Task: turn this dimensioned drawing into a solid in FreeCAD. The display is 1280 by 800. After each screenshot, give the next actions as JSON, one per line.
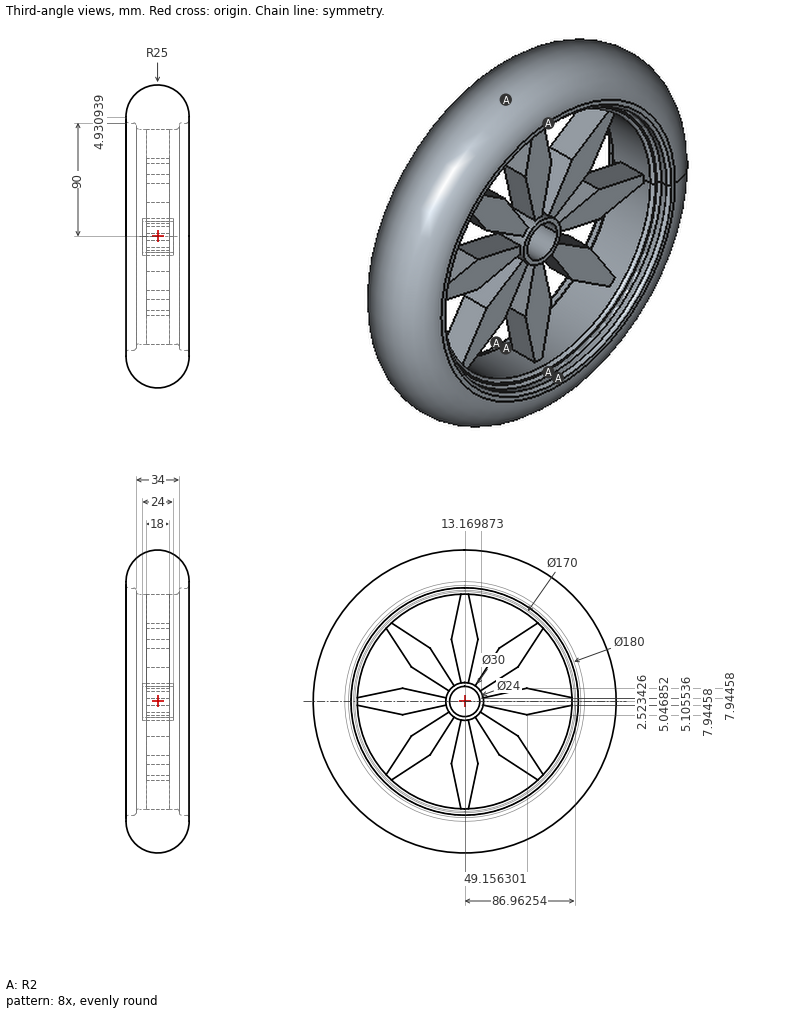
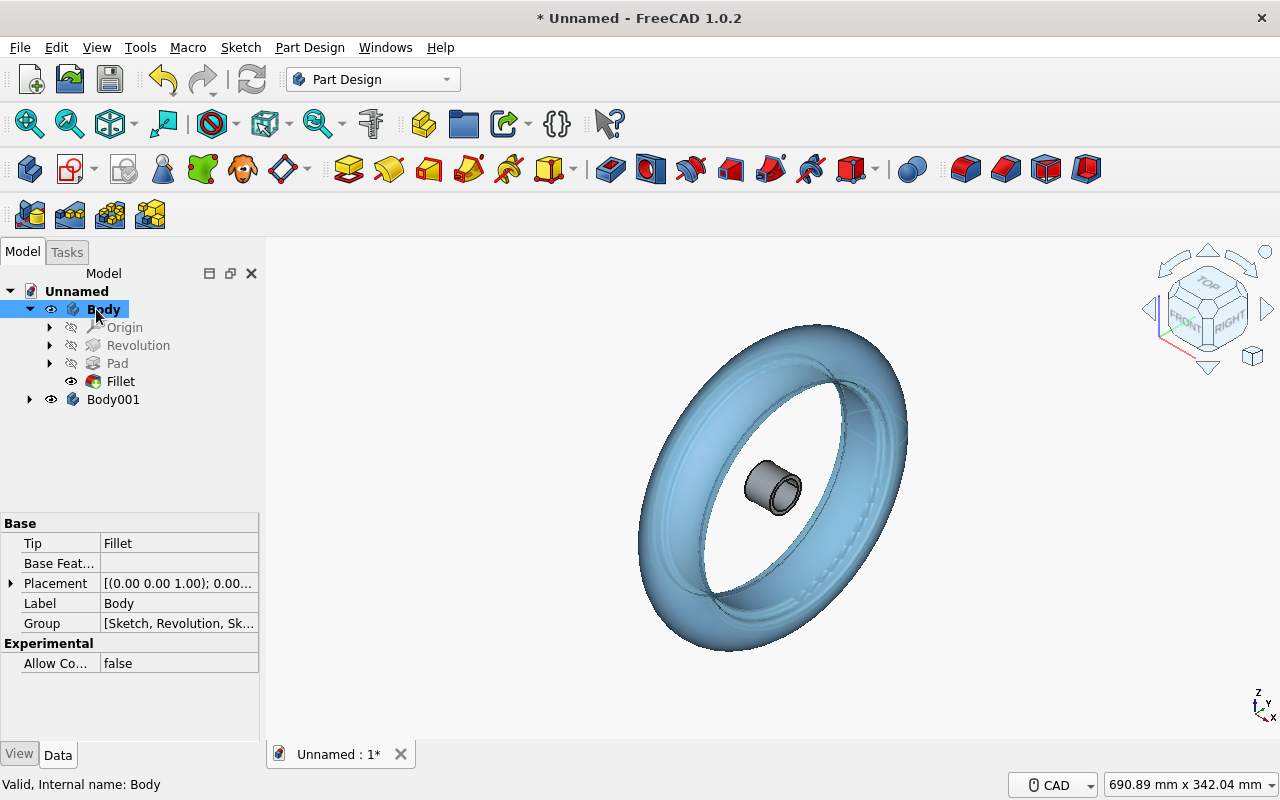
{"action": "left_click", "coordinate": [146, 663]}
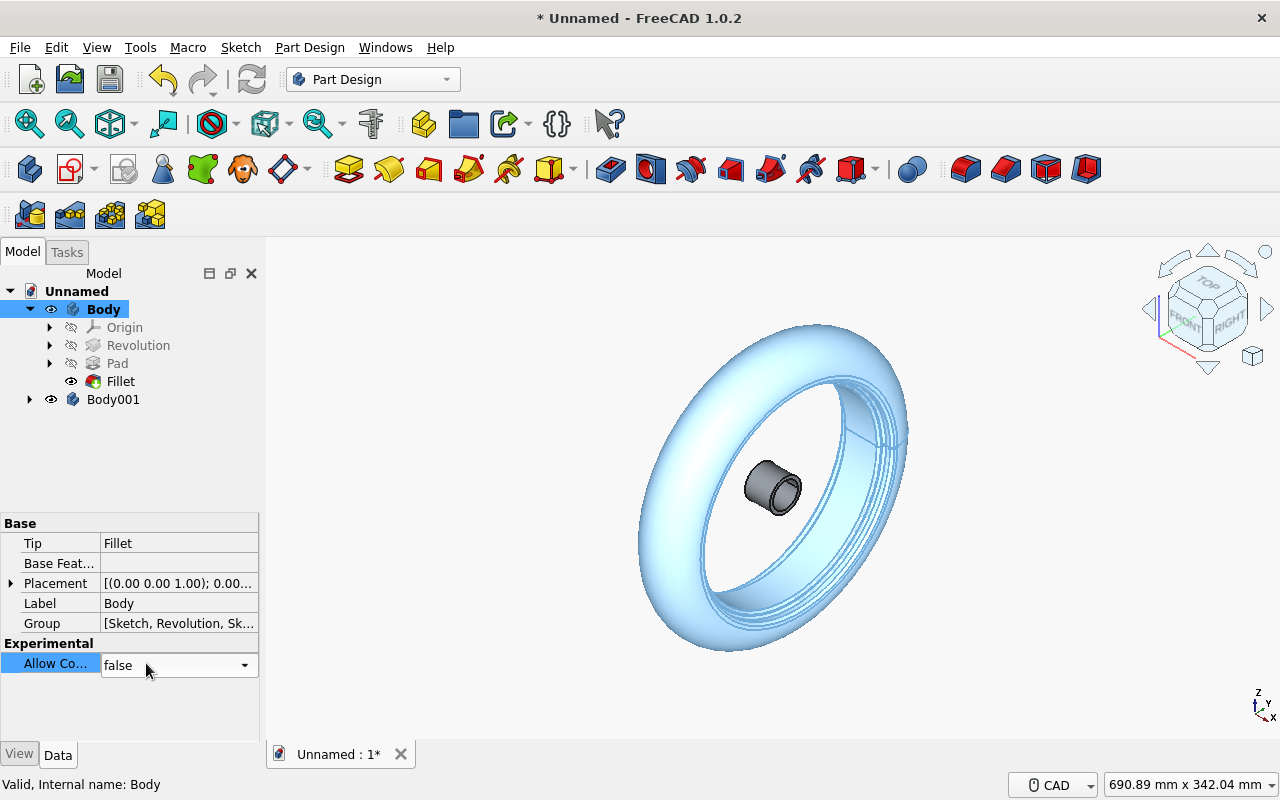
{"action": "left_click", "coordinate": [146, 663]}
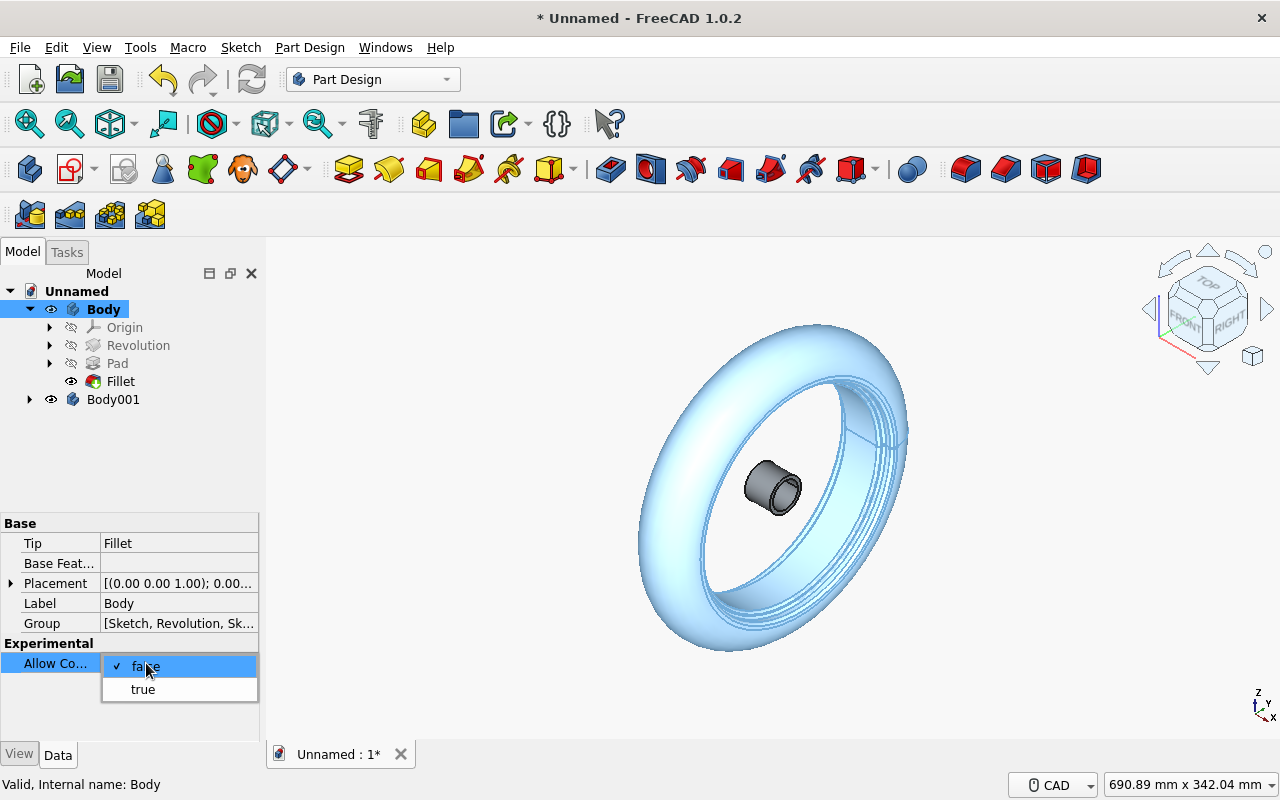
{"action": "left_click", "coordinate": [179, 690]}
{"action": "key", "text": "Return"}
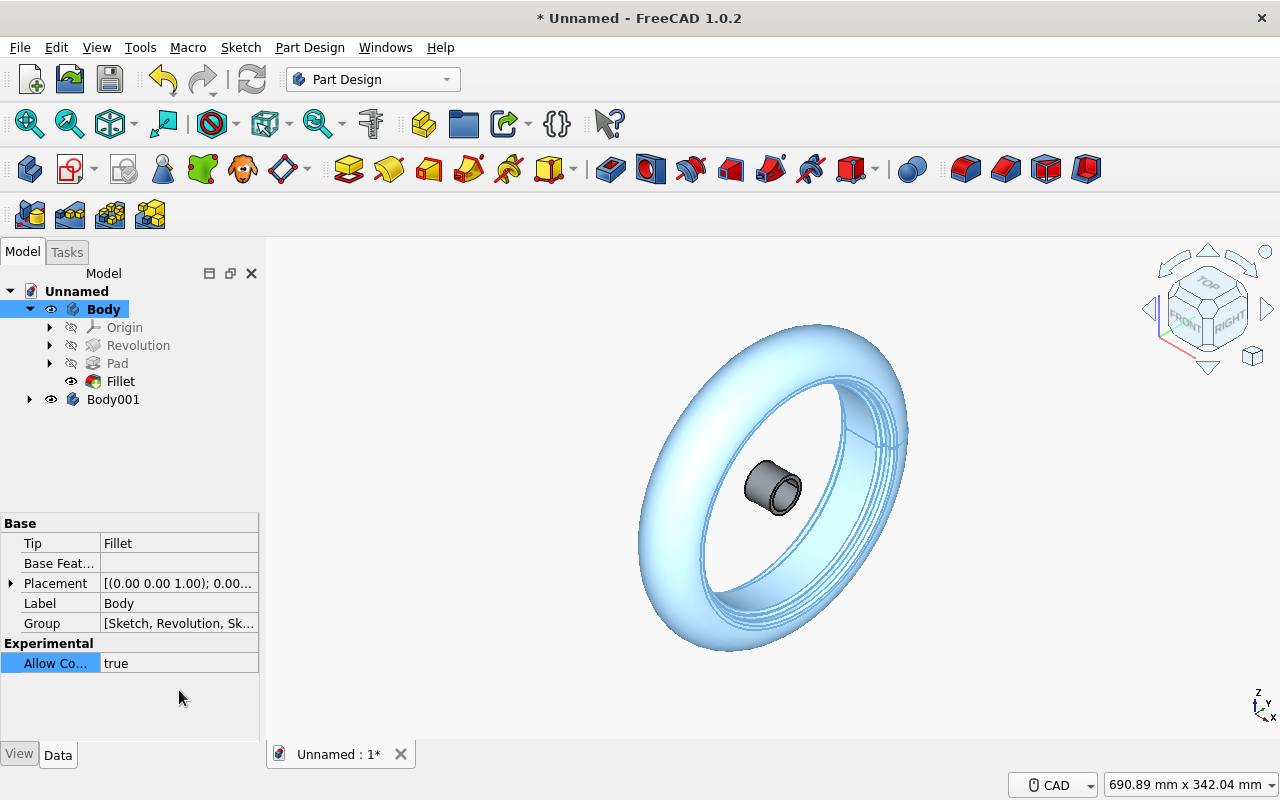
{"action": "left_click", "coordinate": [96, 399]}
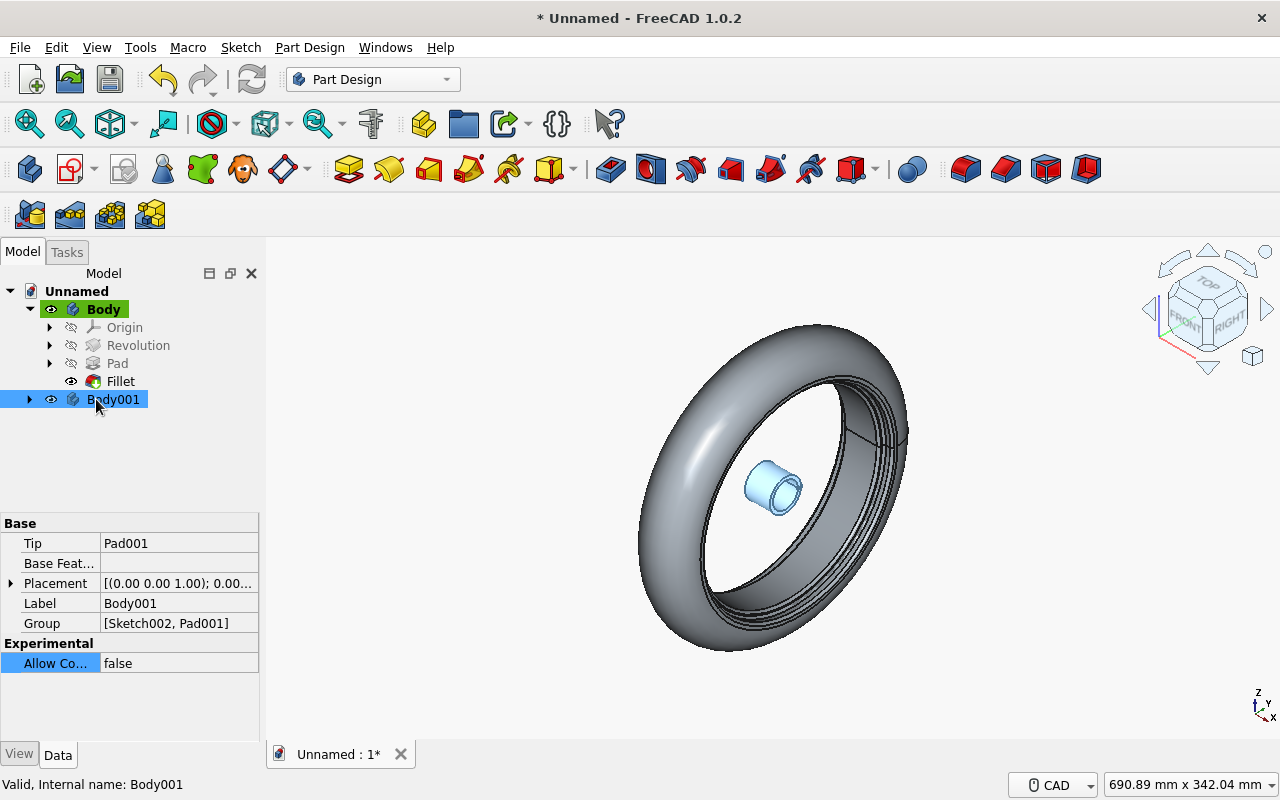
{"action": "left_click", "coordinate": [914, 170]}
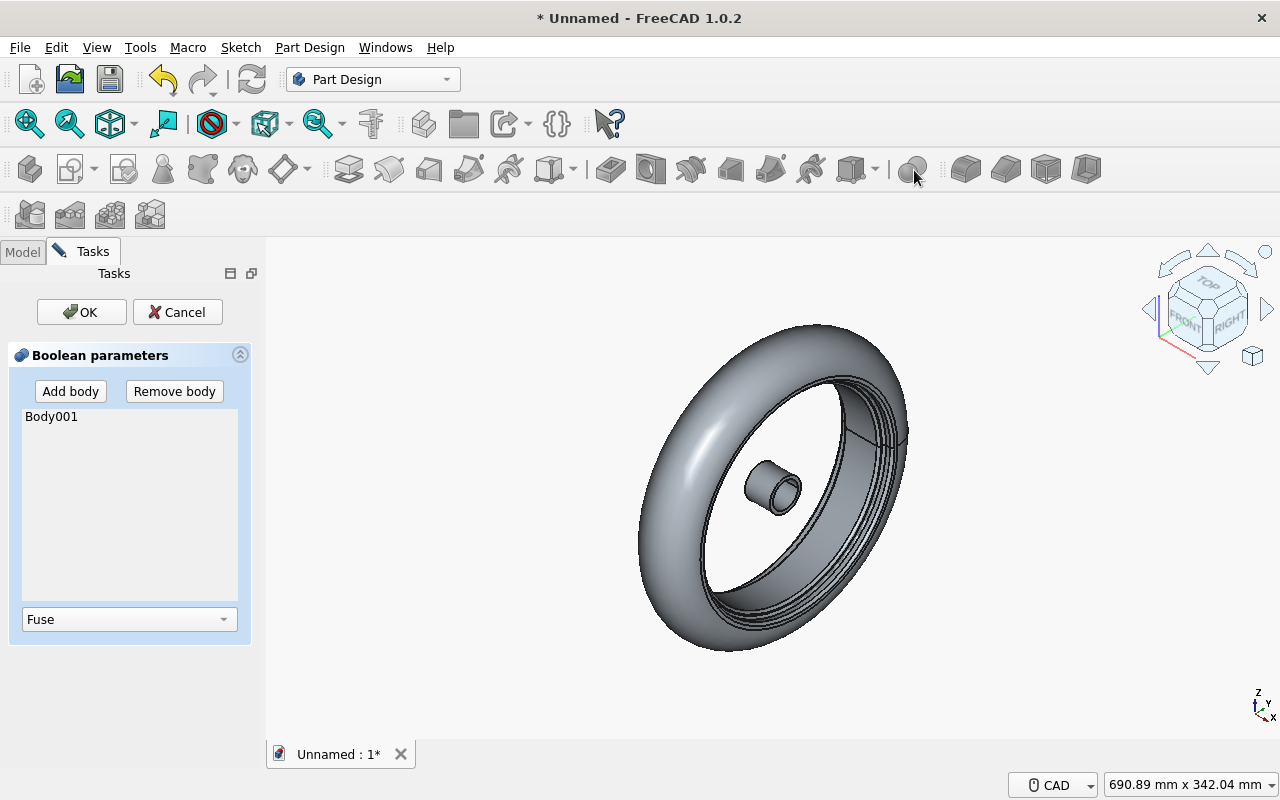
{"action": "left_click", "coordinate": [82, 312]}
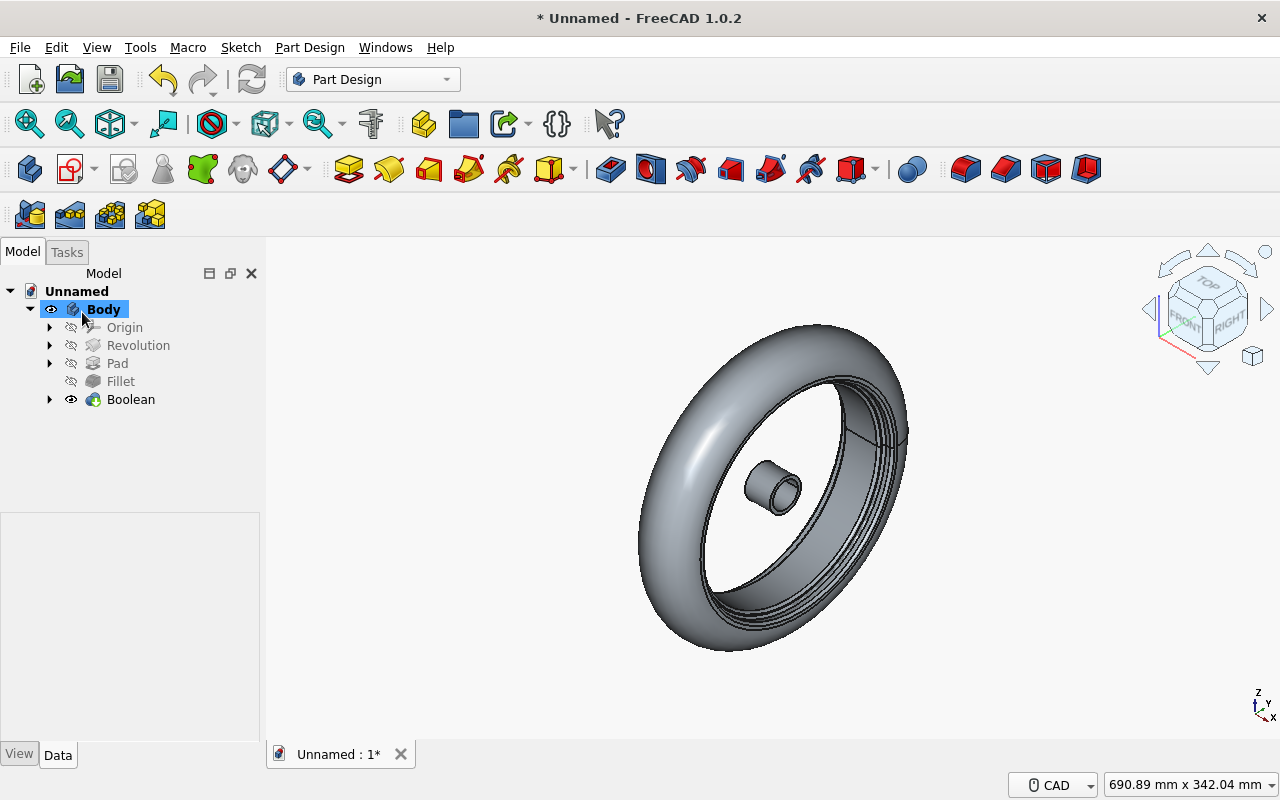
{"action": "left_click", "coordinate": [70, 170]}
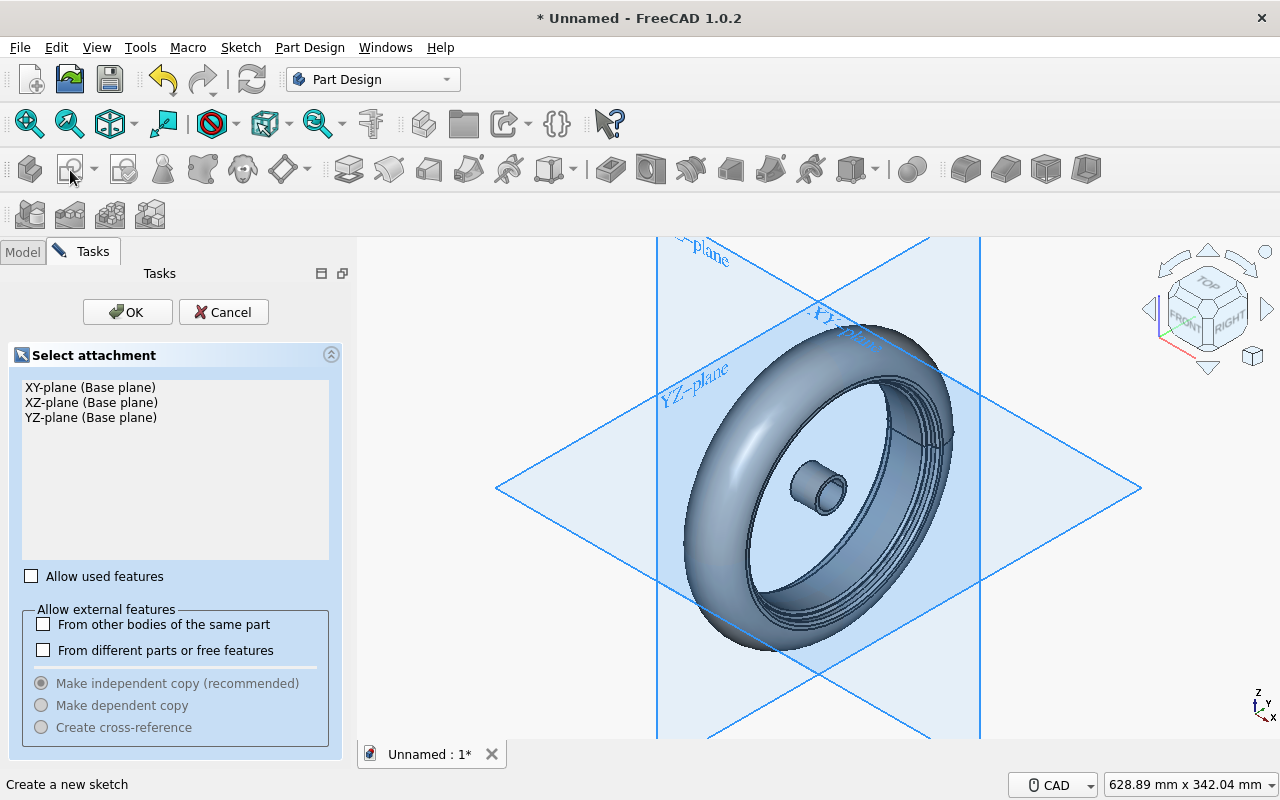
{"action": "left_click", "coordinate": [82, 418]}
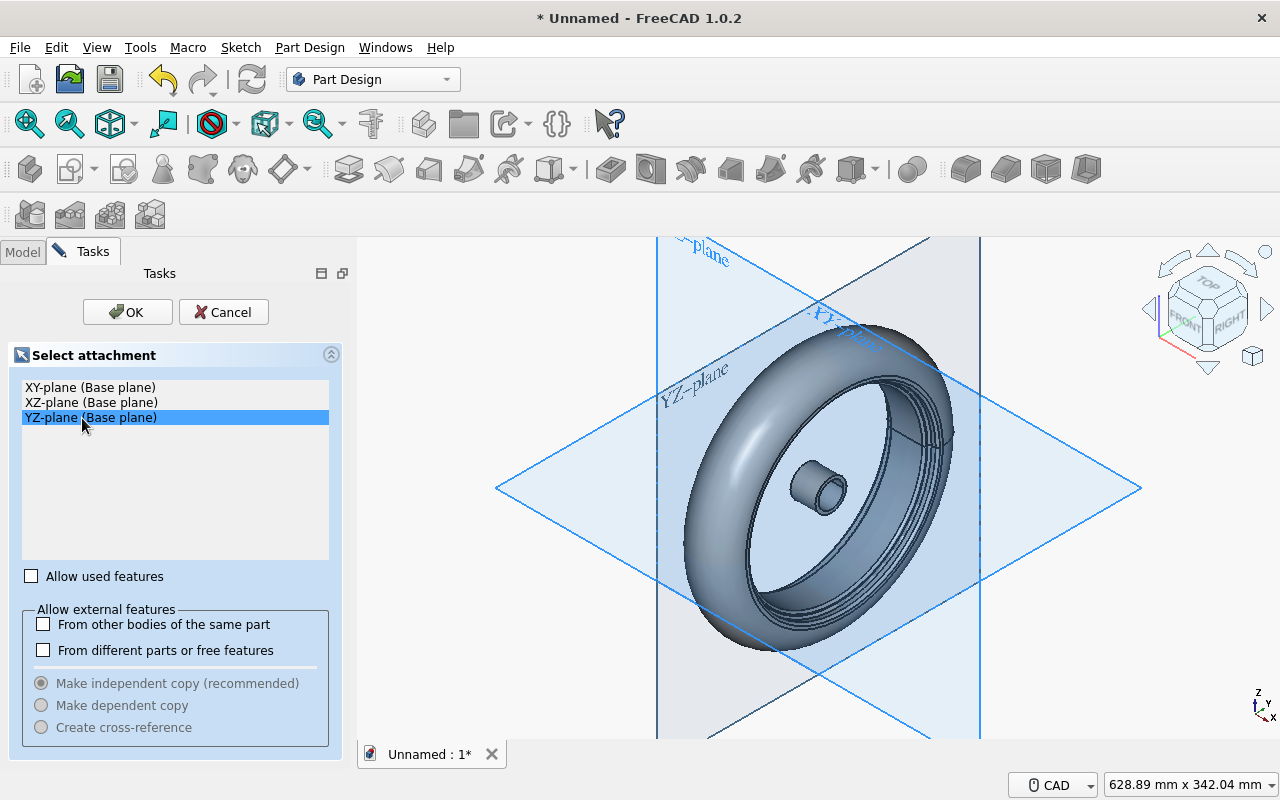
{"action": "left_click", "coordinate": [128, 312]}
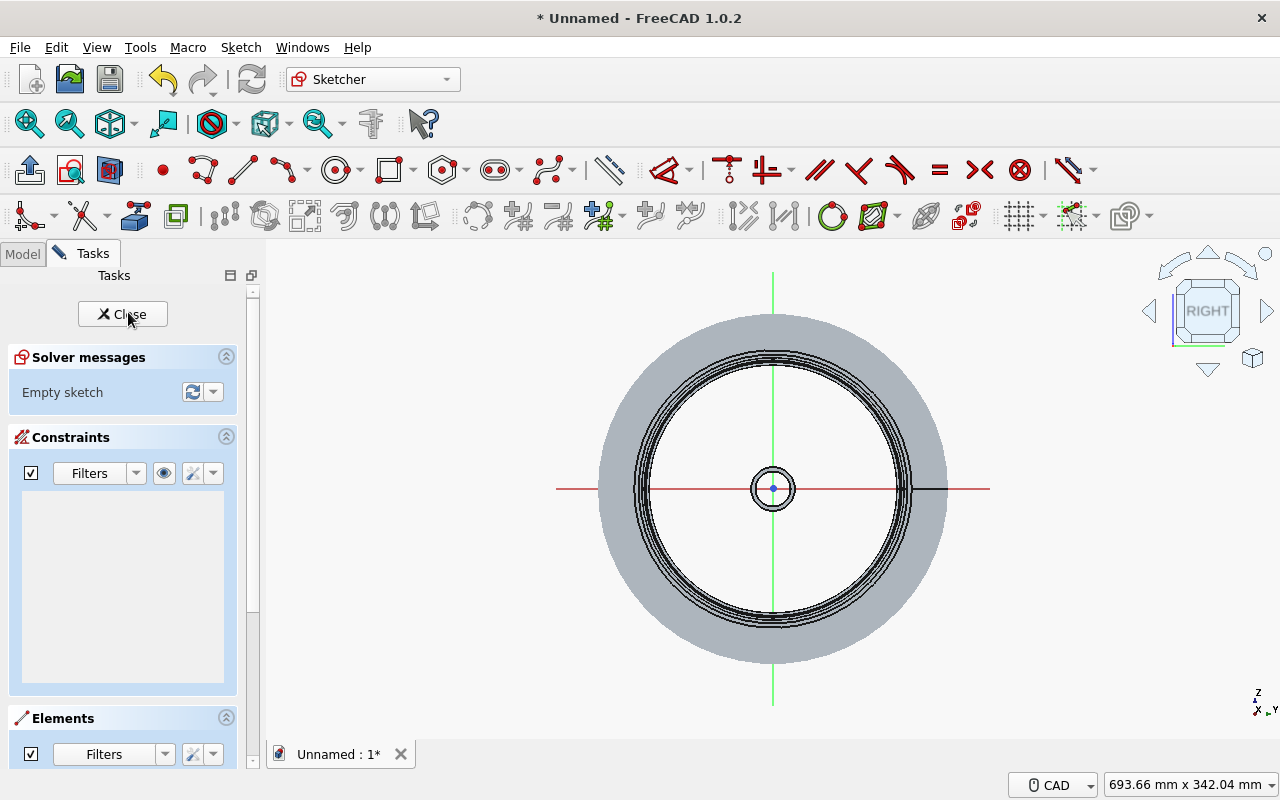
{"action": "key", "text": "q s"}